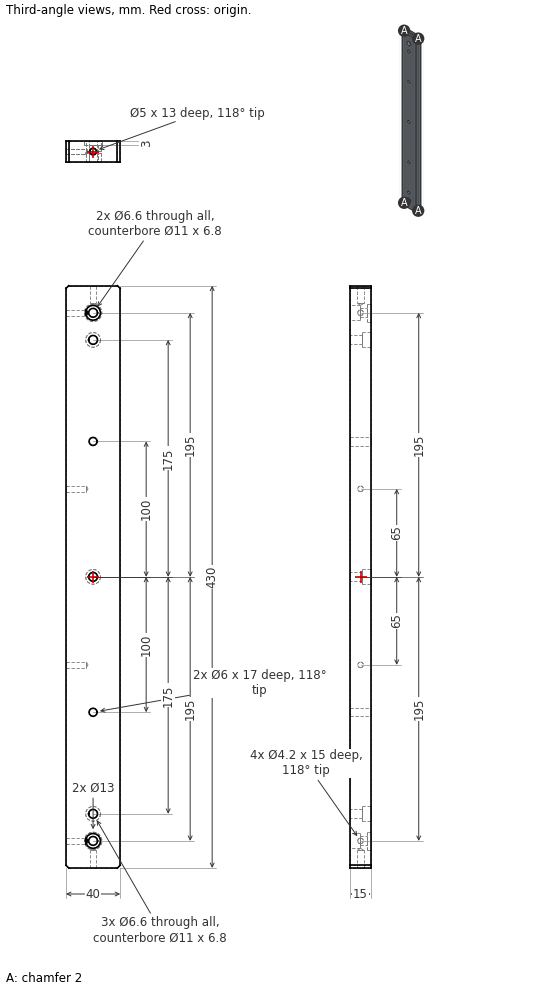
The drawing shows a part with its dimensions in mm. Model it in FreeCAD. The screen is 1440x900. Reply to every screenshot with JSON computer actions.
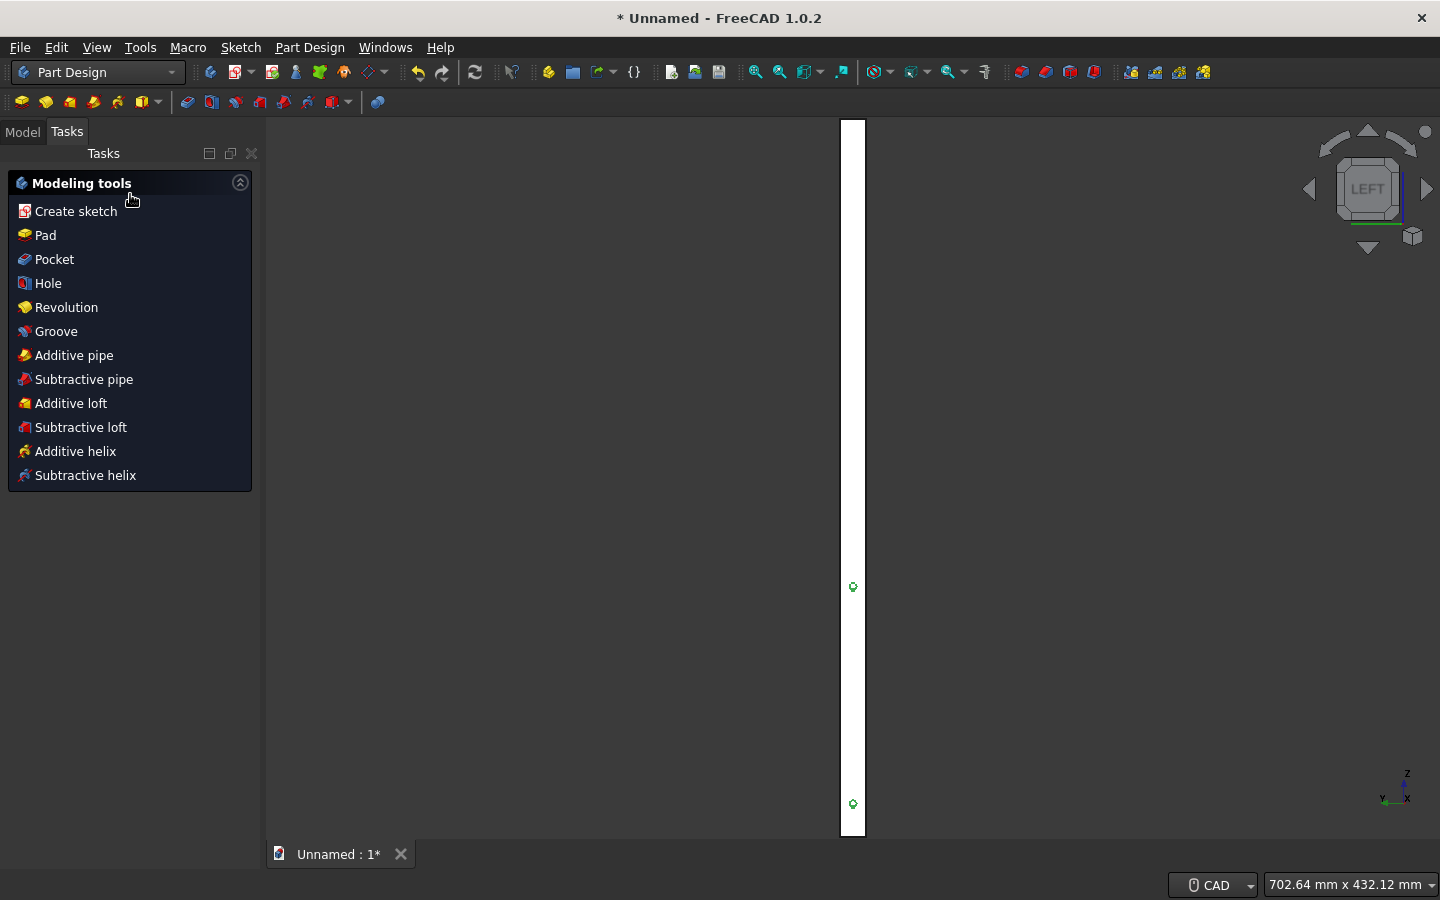
{"action": "left_click", "coordinate": [212, 102]}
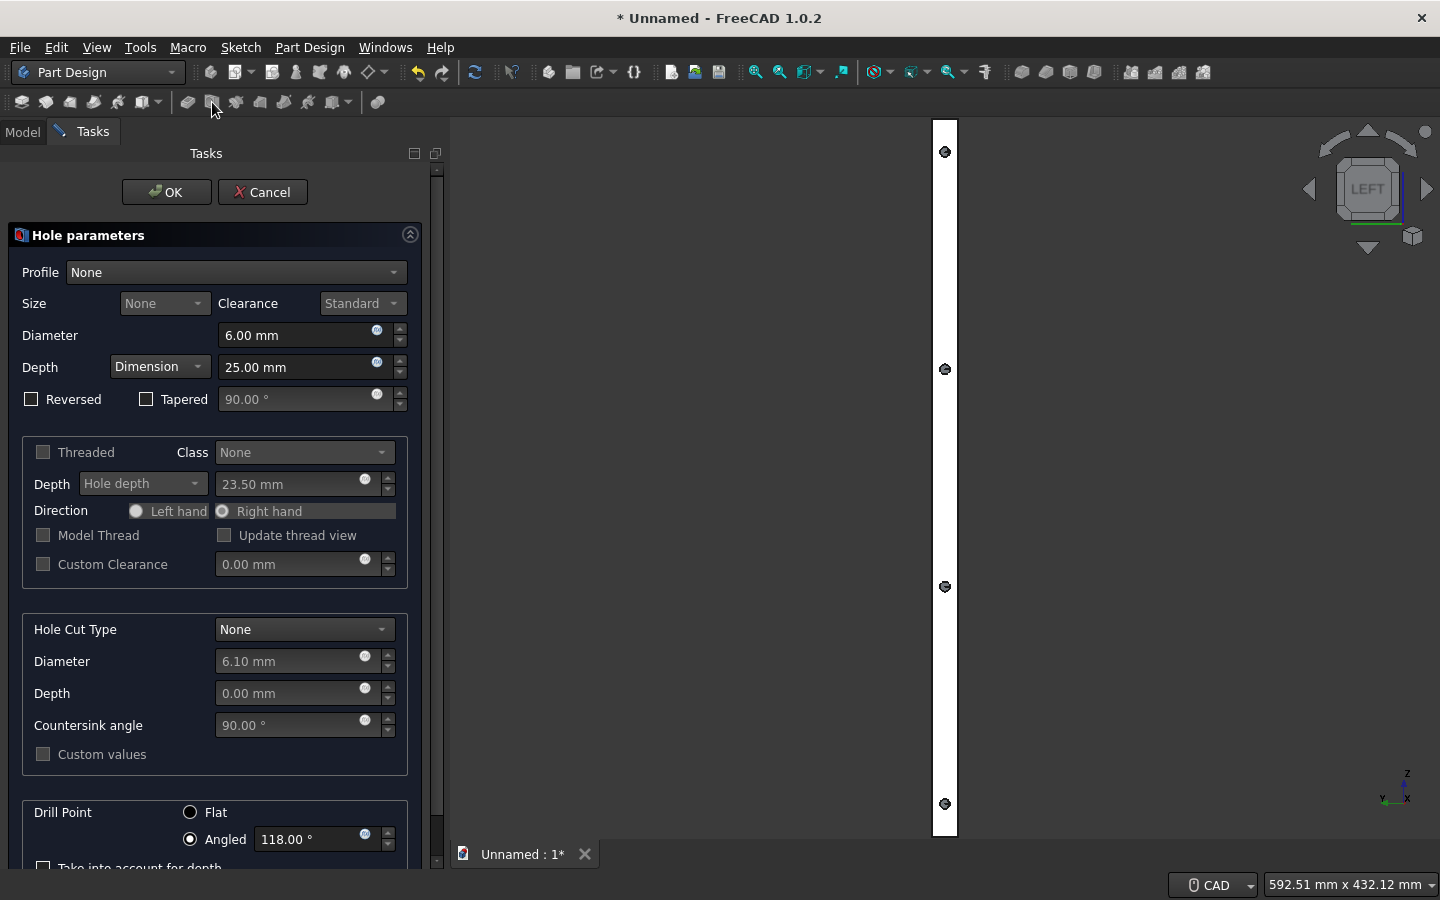
{"action": "triple_click", "coordinate": [305, 335]}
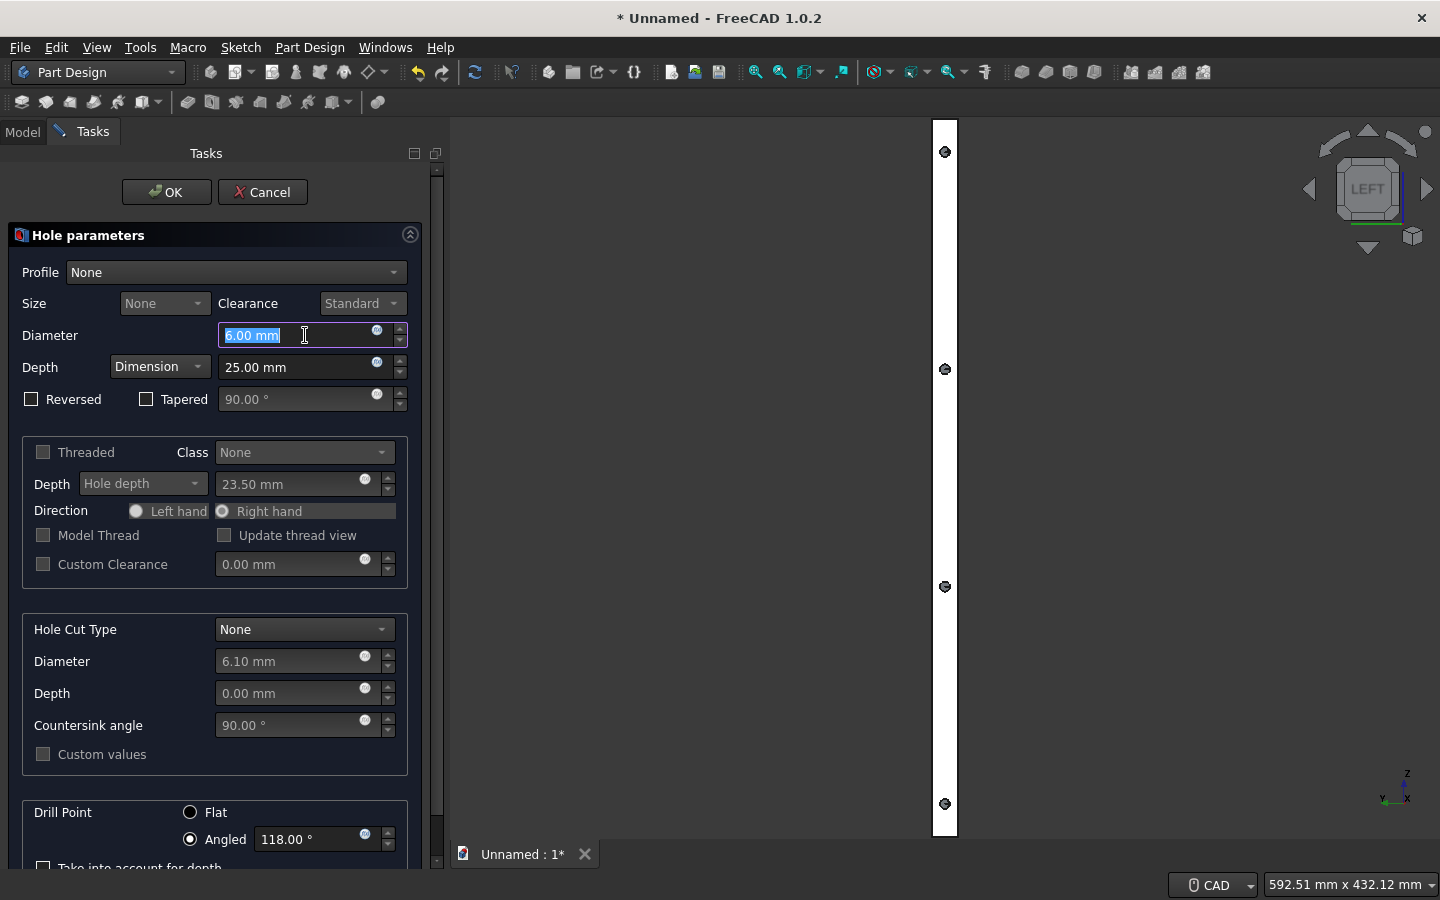
{"action": "type", "text": "4.2"}
{"action": "key", "text": "Tab"}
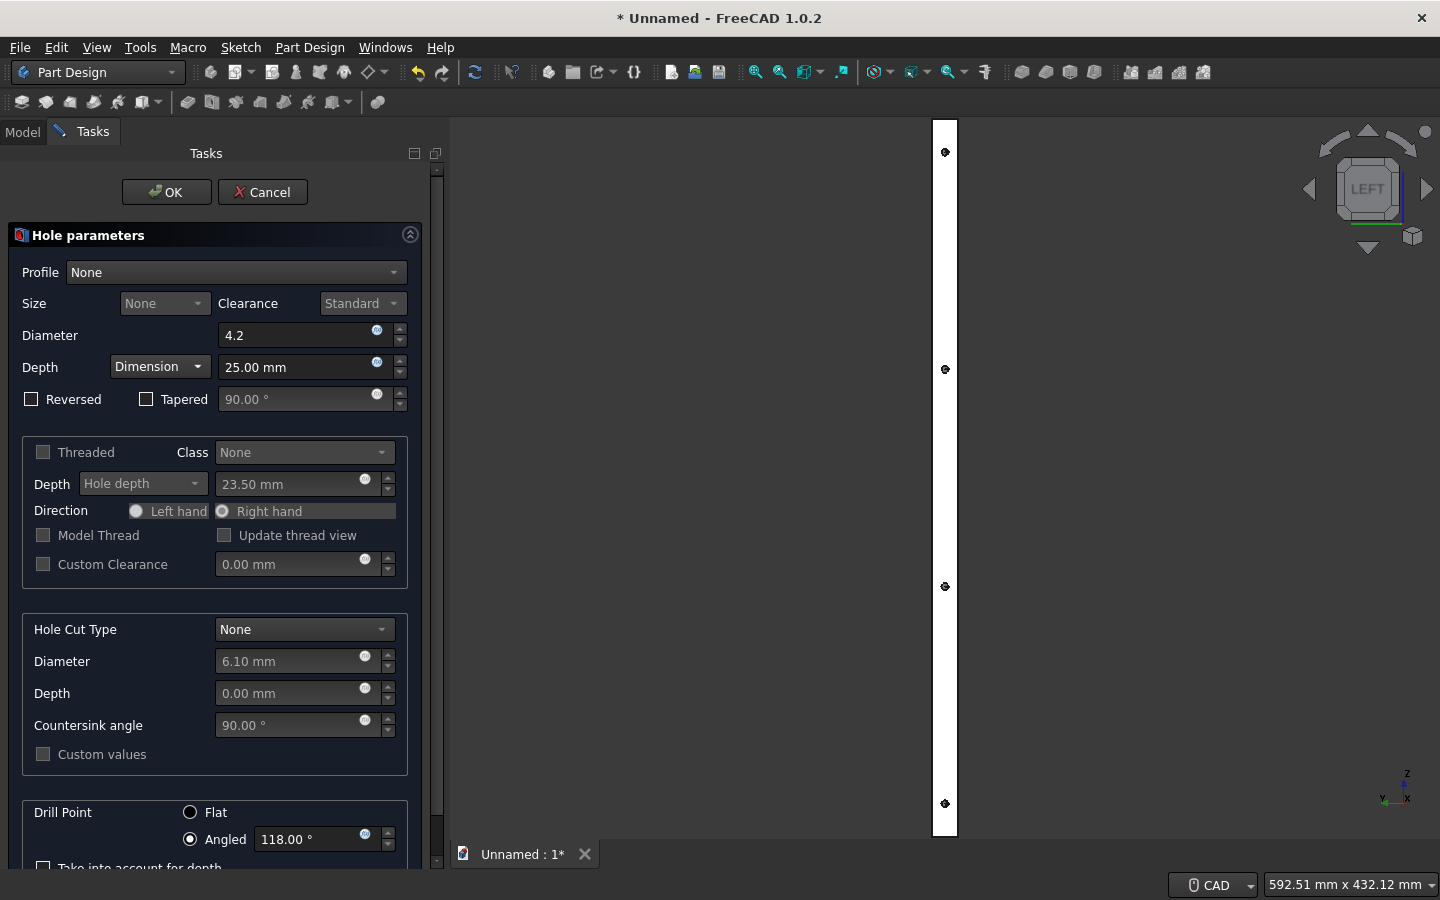
{"action": "triple_click", "coordinate": [305, 367]}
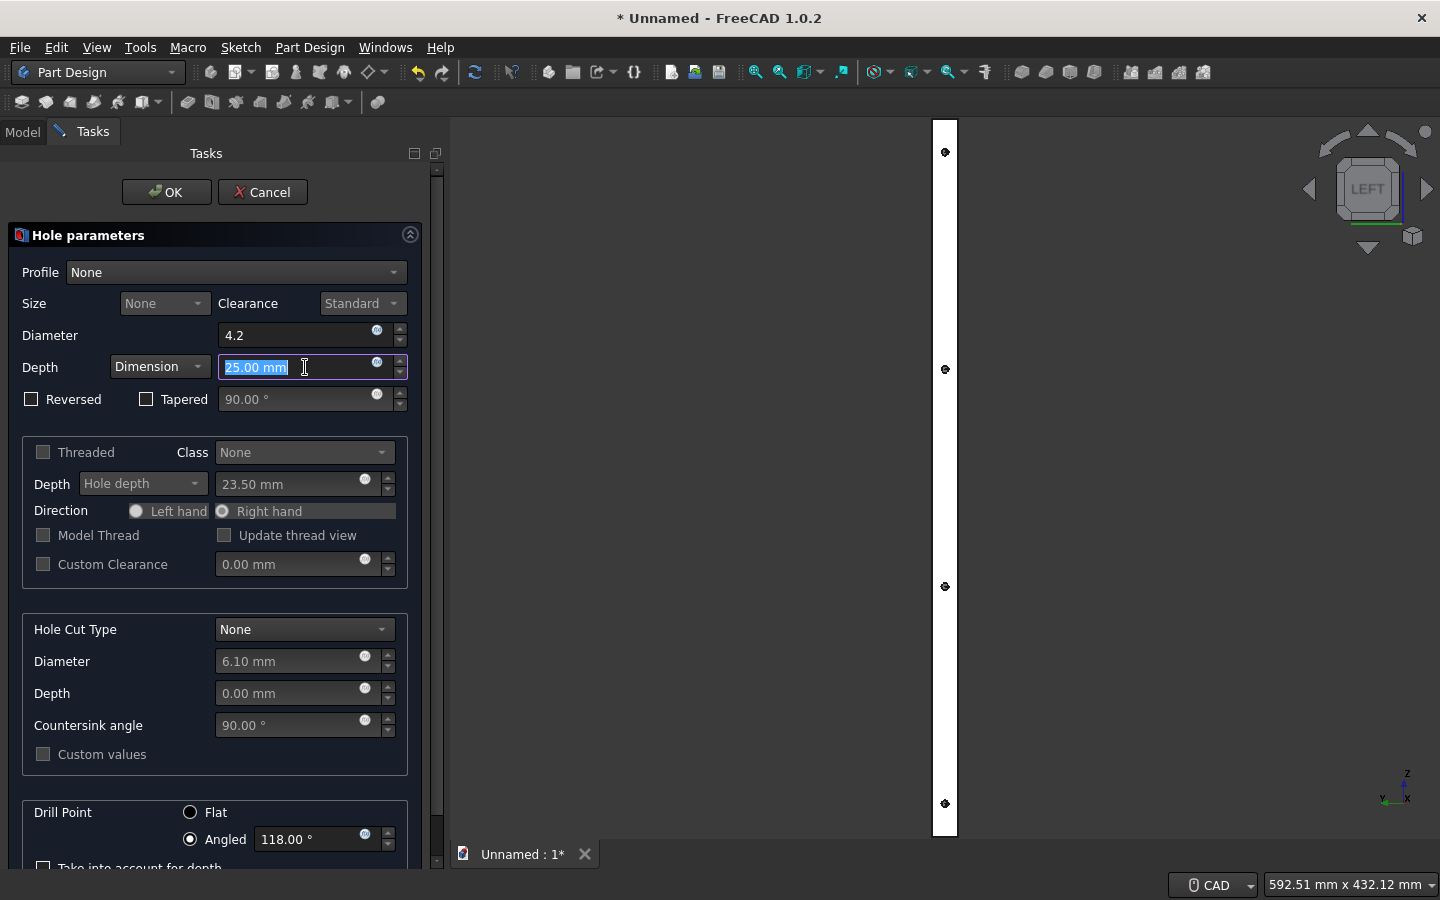
{"action": "type", "text": "15"}
{"action": "key", "text": "Tab"}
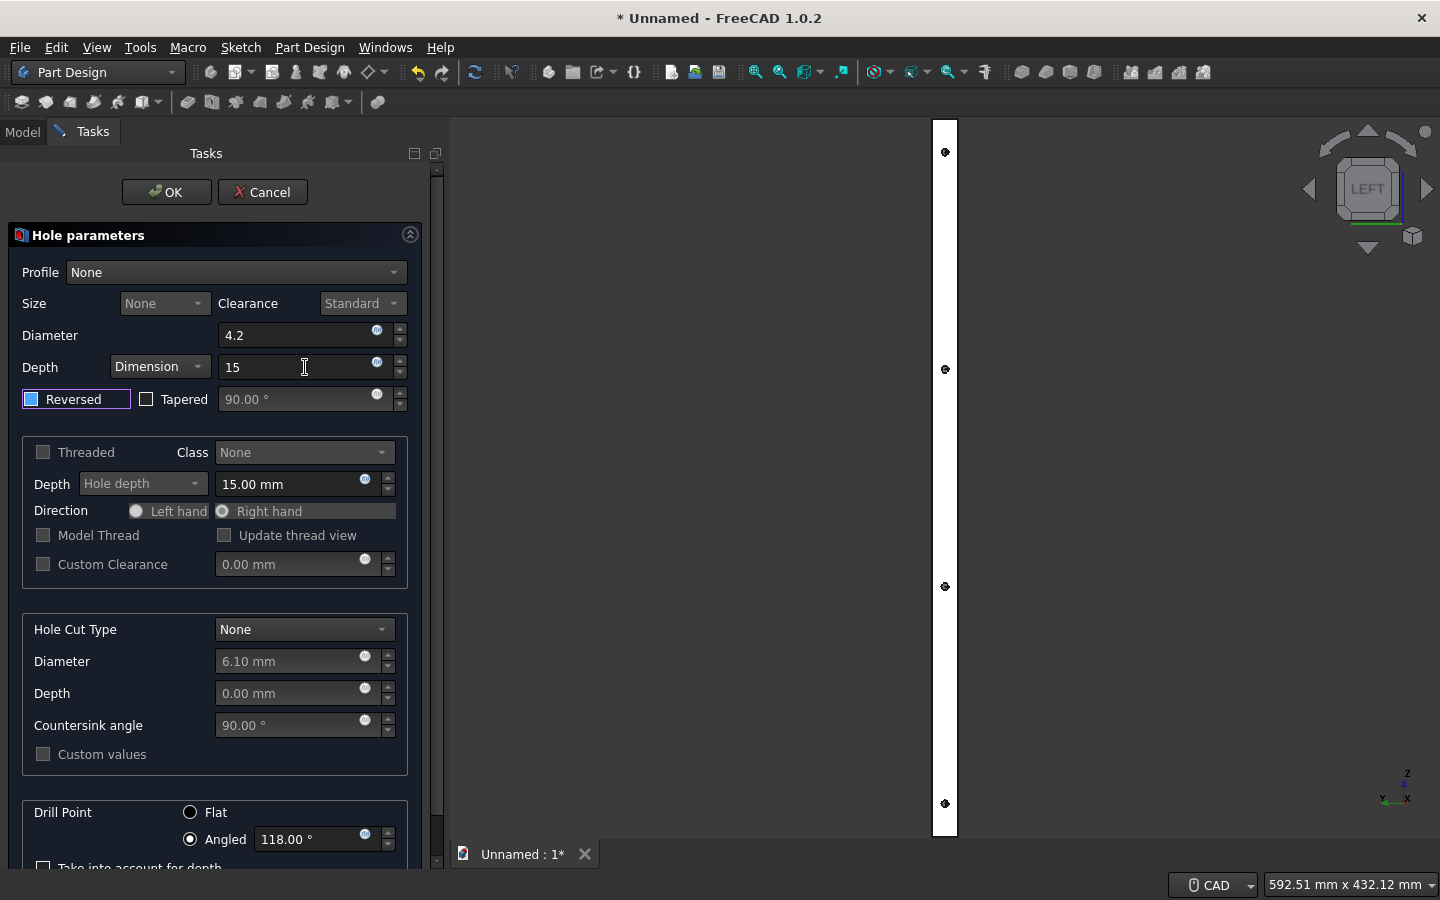
{"action": "left_click", "coordinate": [167, 192]}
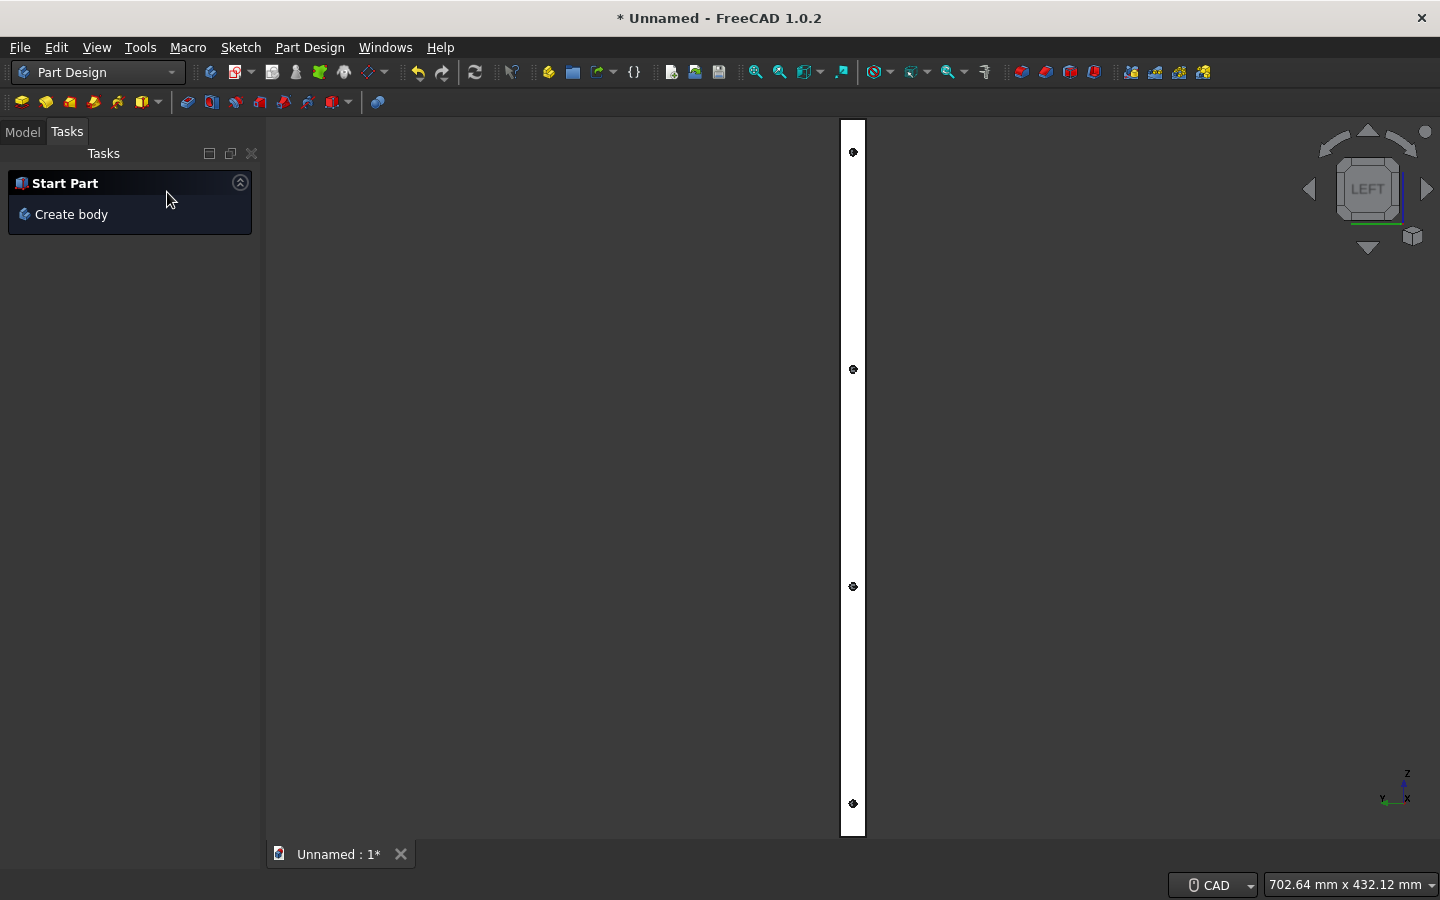
{"action": "key", "text": "0"}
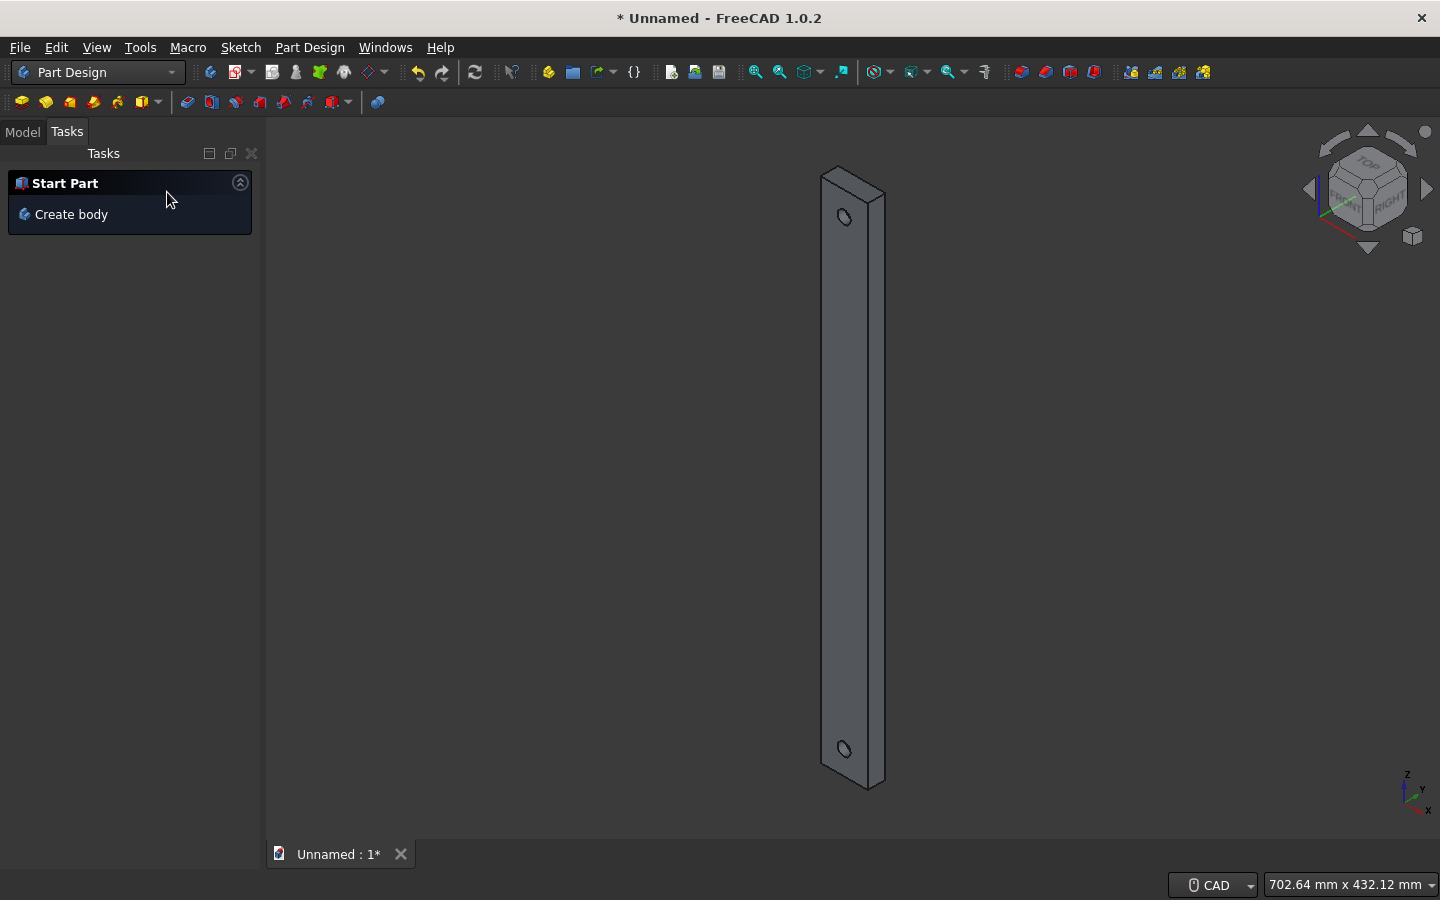
{"action": "left_click", "coordinate": [877, 197]}